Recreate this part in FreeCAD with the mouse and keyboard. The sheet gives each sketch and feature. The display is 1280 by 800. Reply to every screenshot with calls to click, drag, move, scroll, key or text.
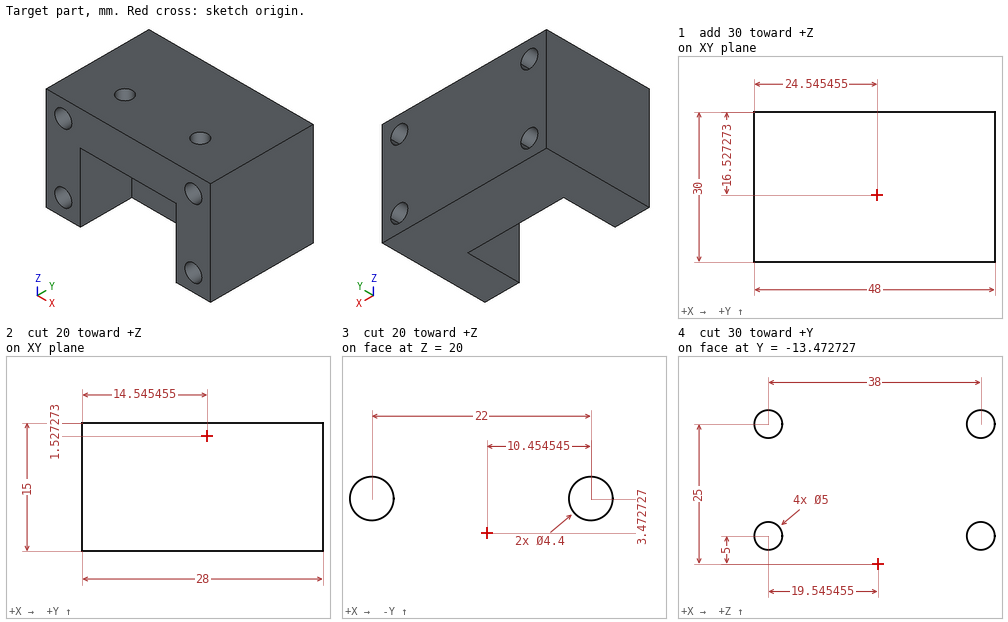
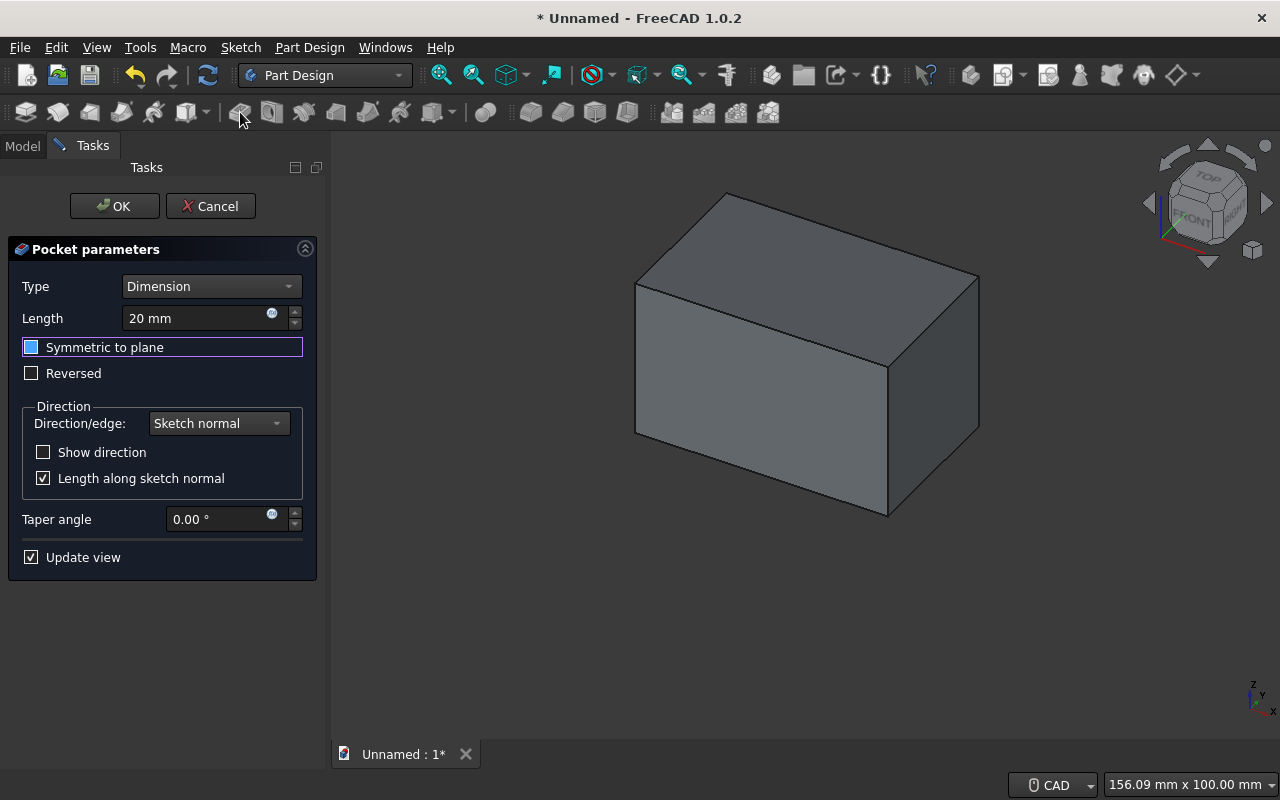
click(30, 373)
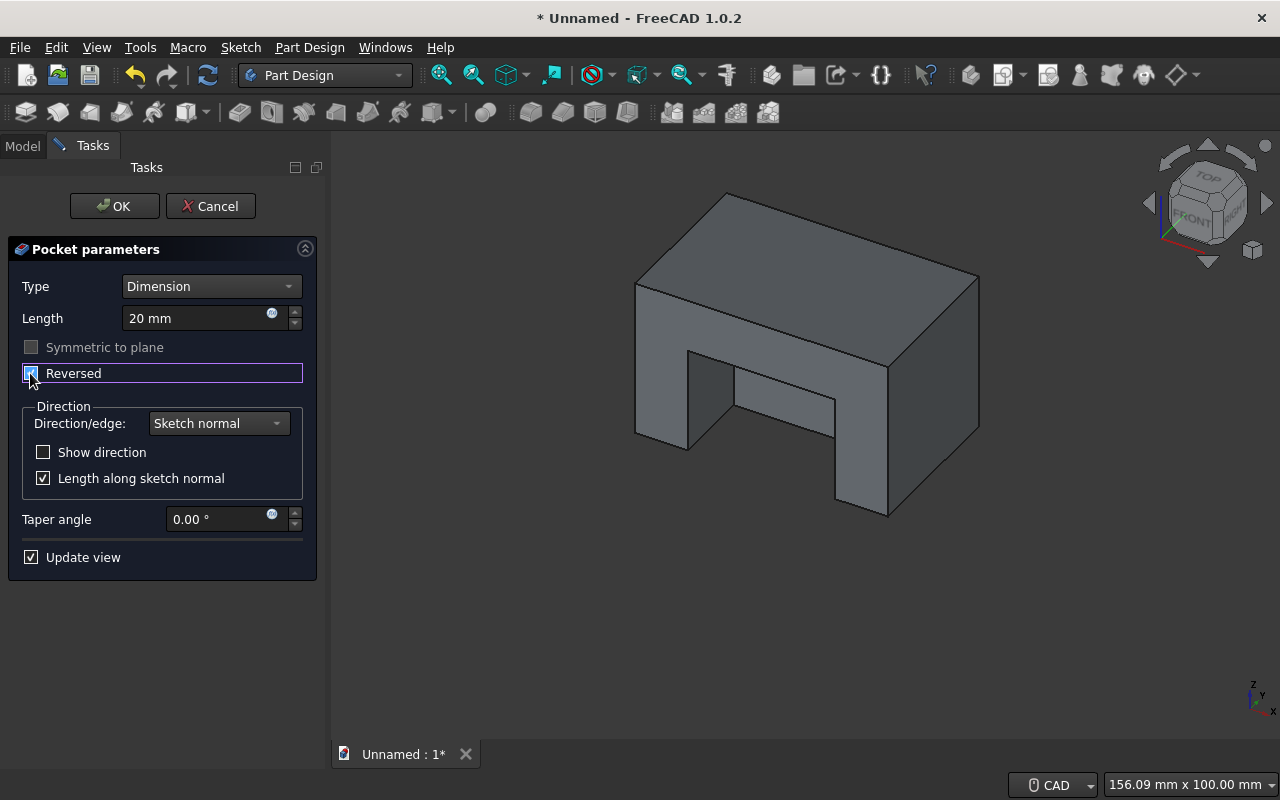
click(115, 206)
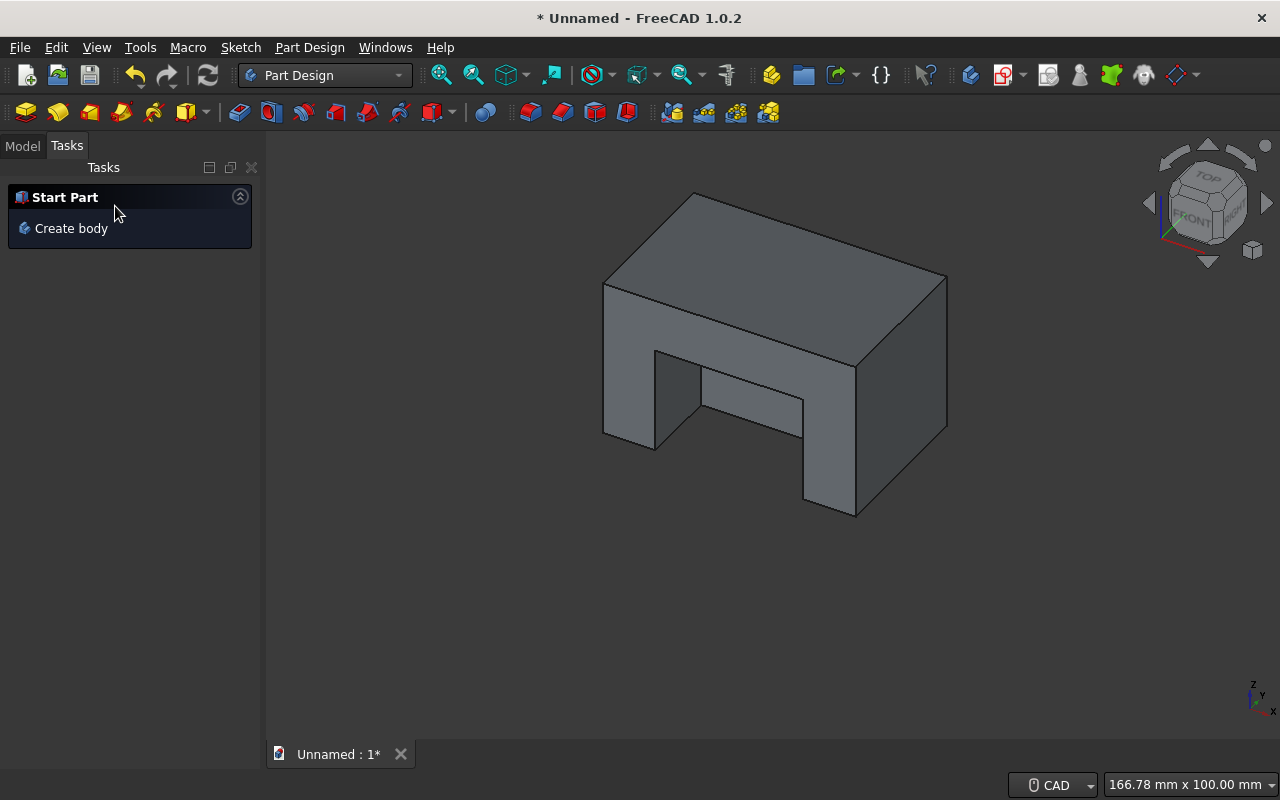
key(5)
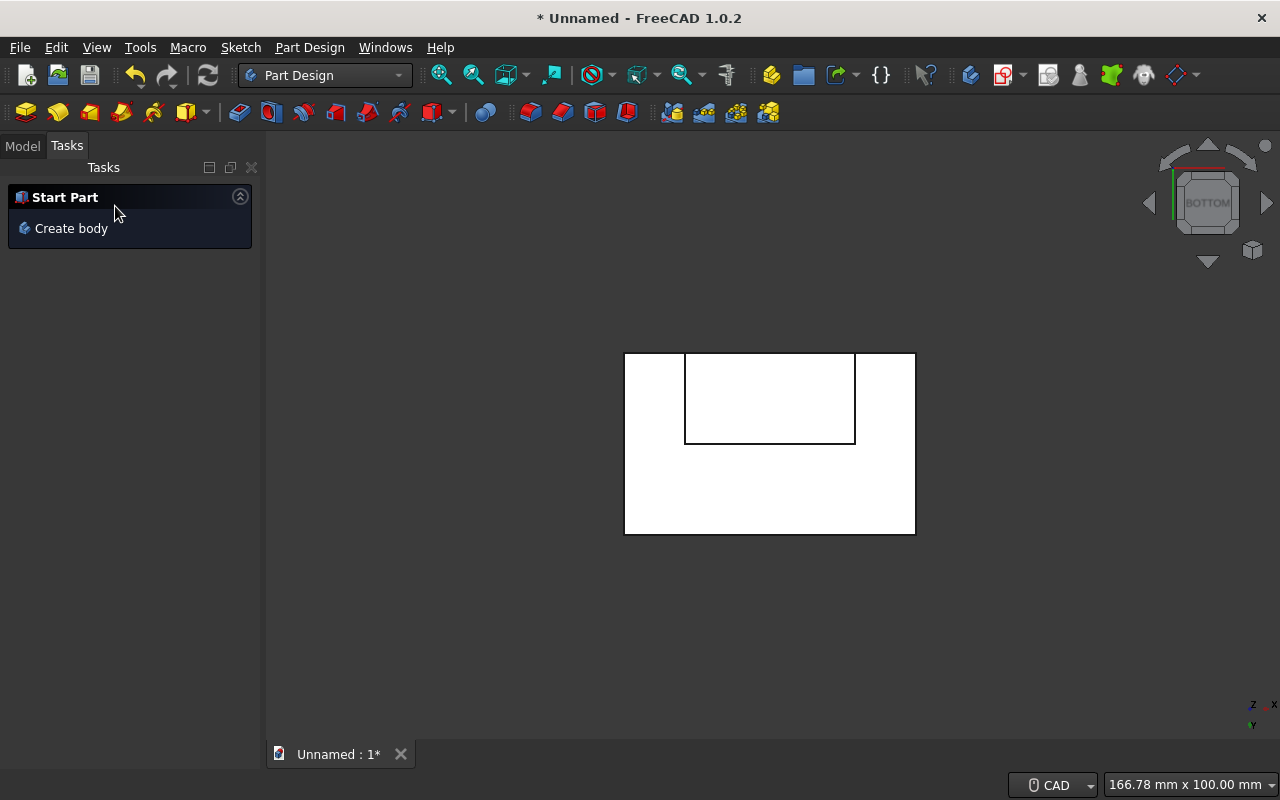
click(442, 76)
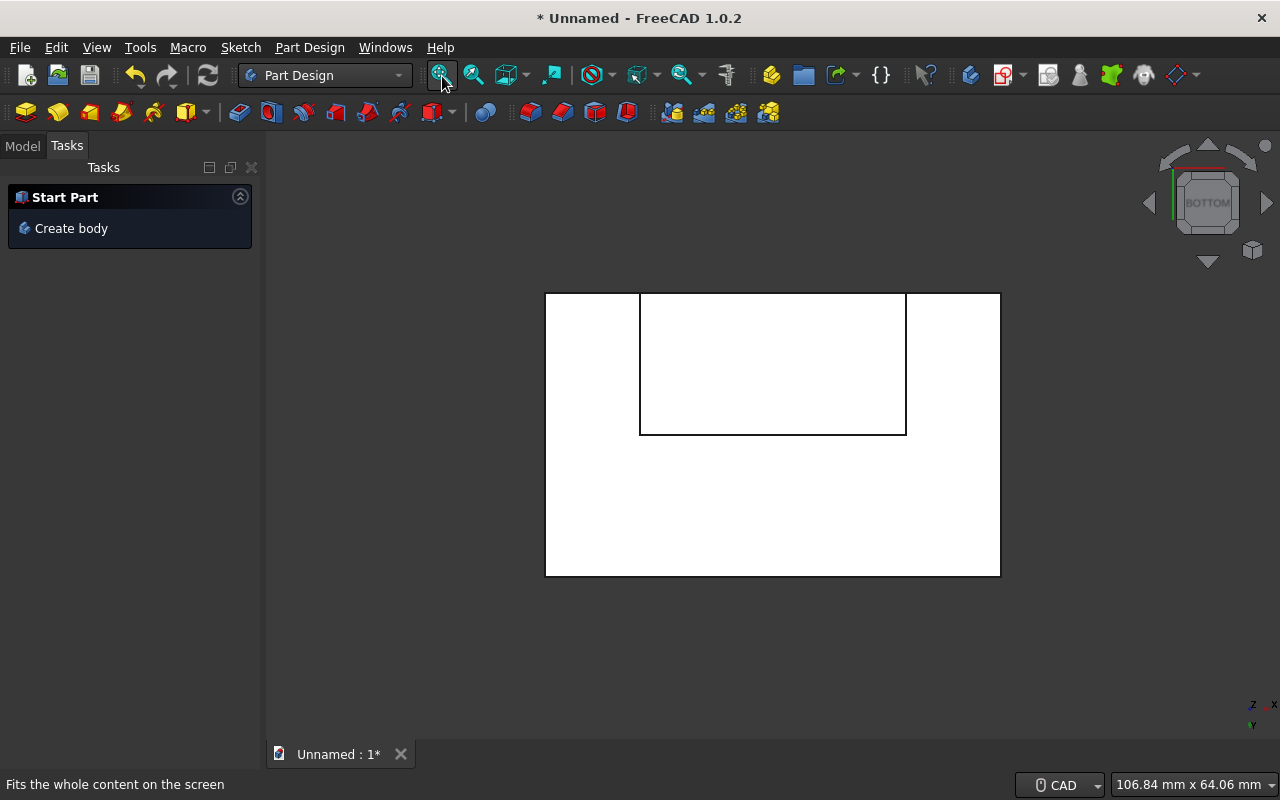
click(811, 363)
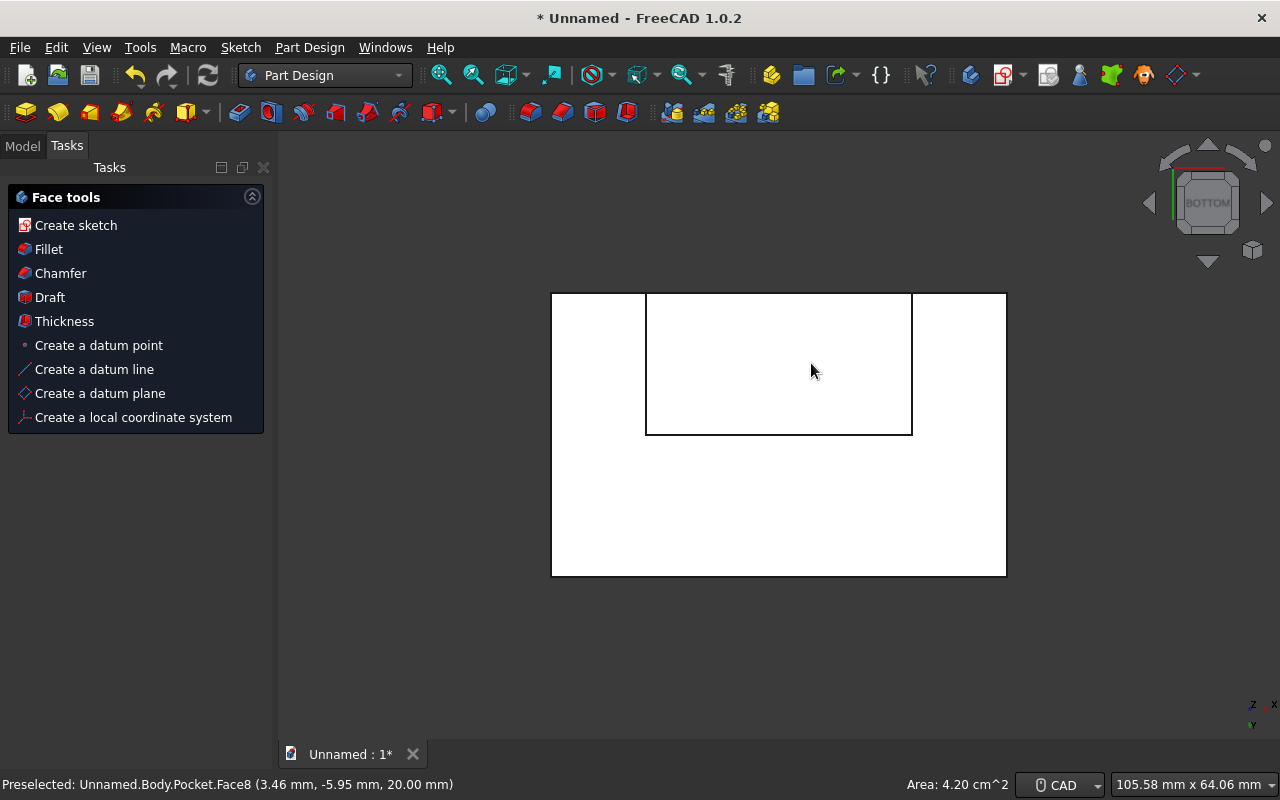
click(1004, 76)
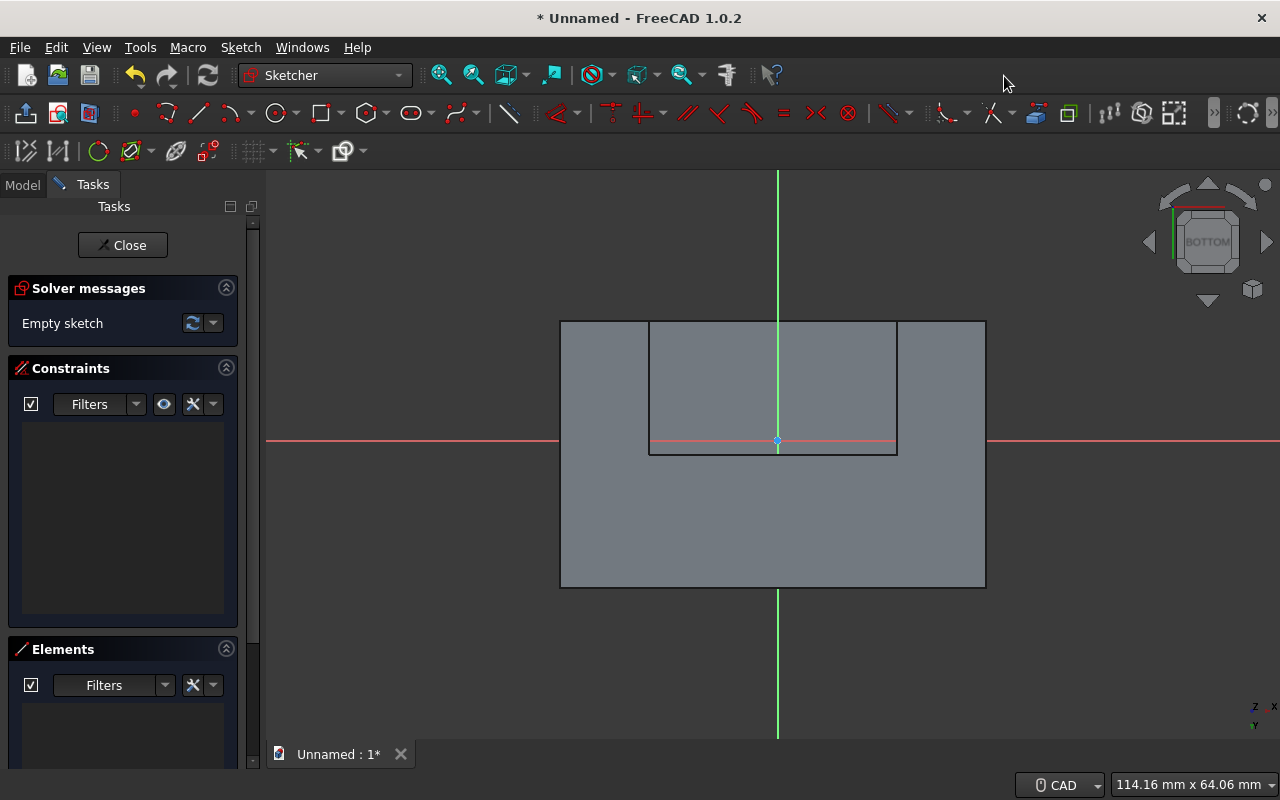
scroll(813, 393, up, 5)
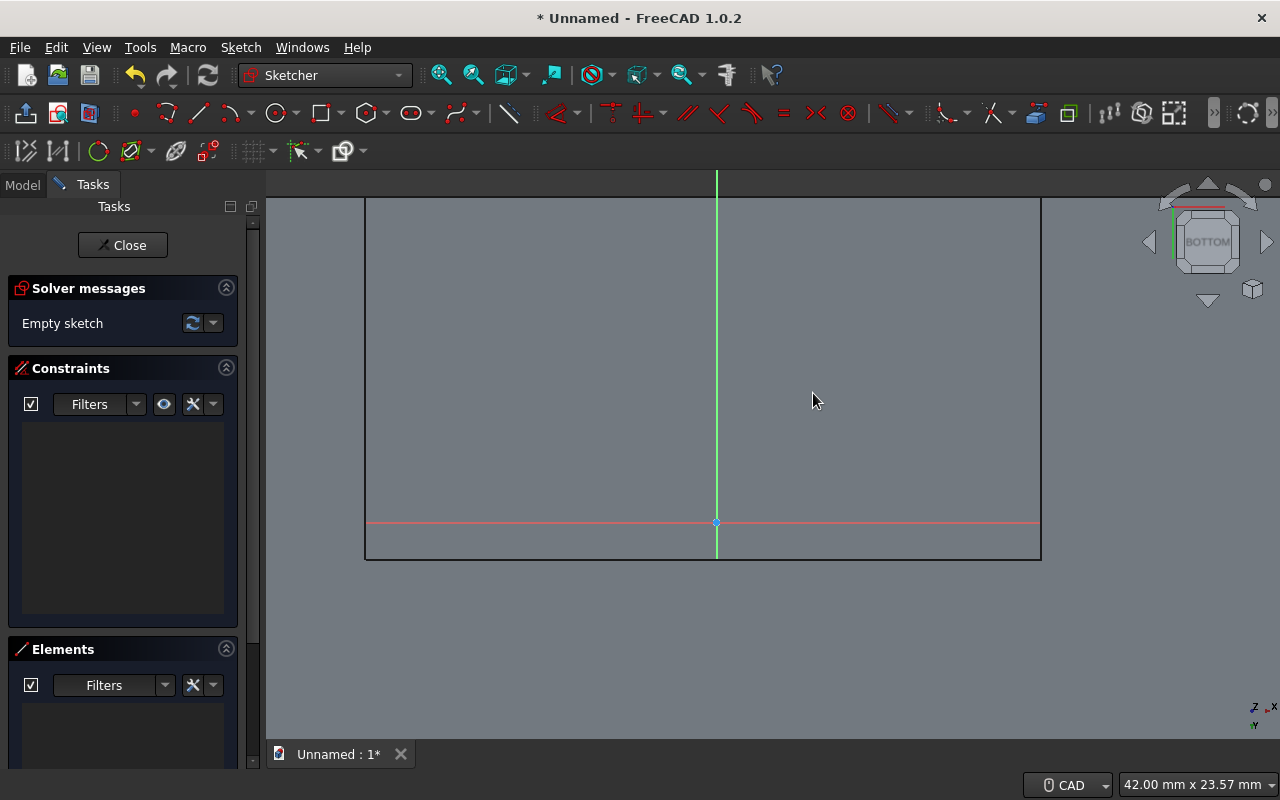
click(276, 114)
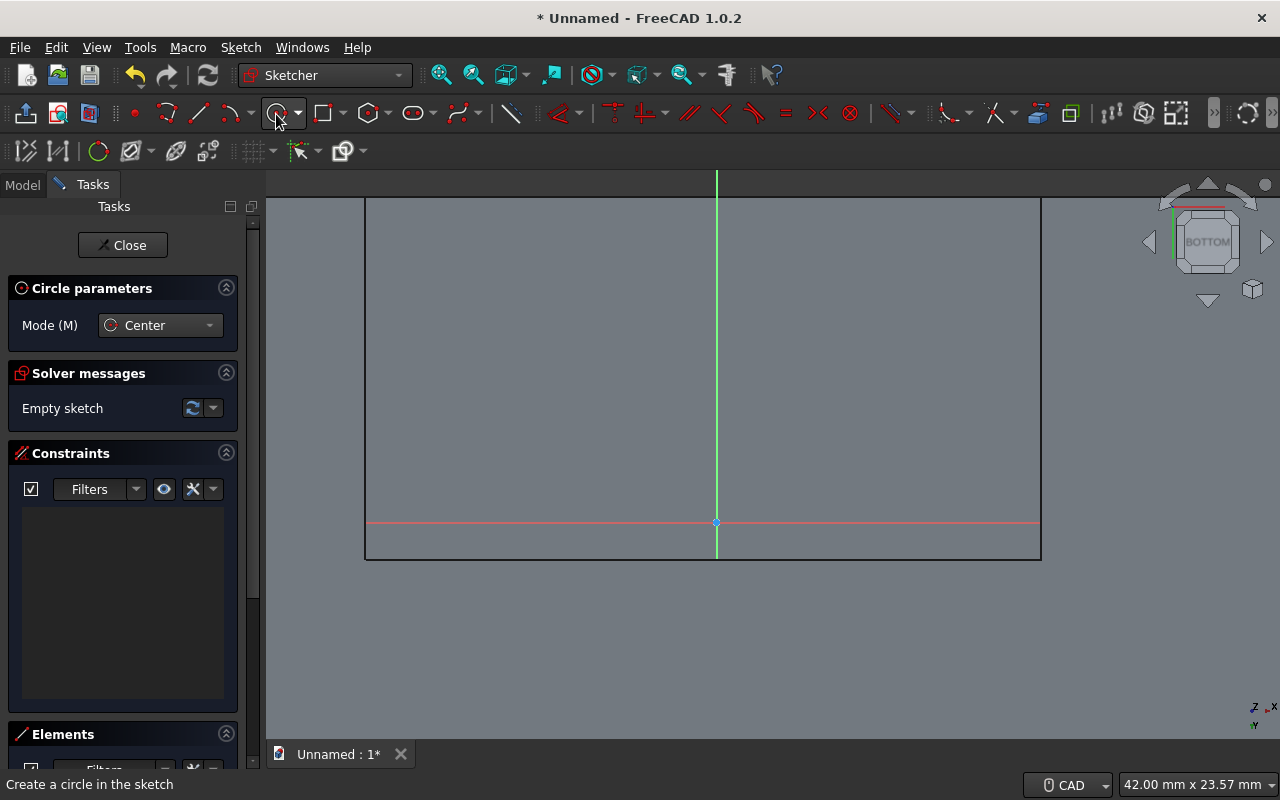
click(969, 439)
click(1006, 401)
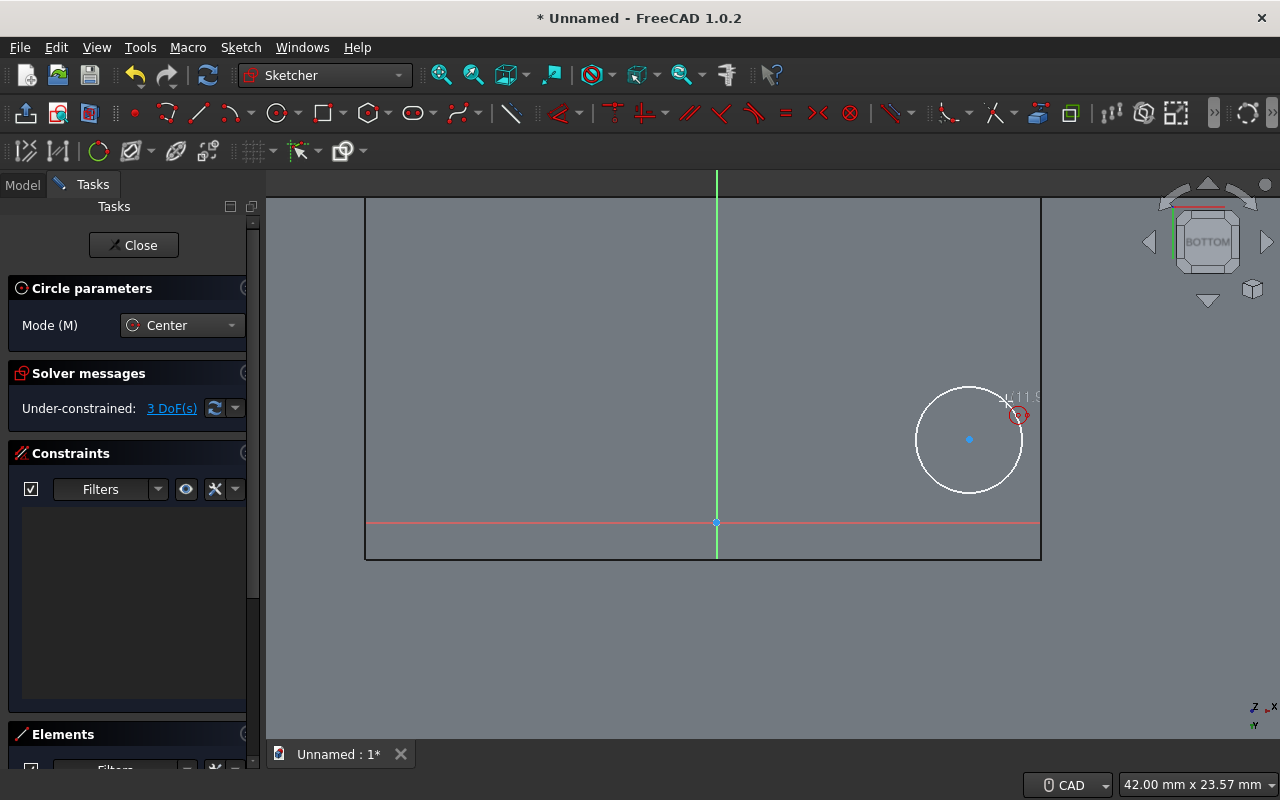
click(438, 439)
click(475, 401)
key(Escape)